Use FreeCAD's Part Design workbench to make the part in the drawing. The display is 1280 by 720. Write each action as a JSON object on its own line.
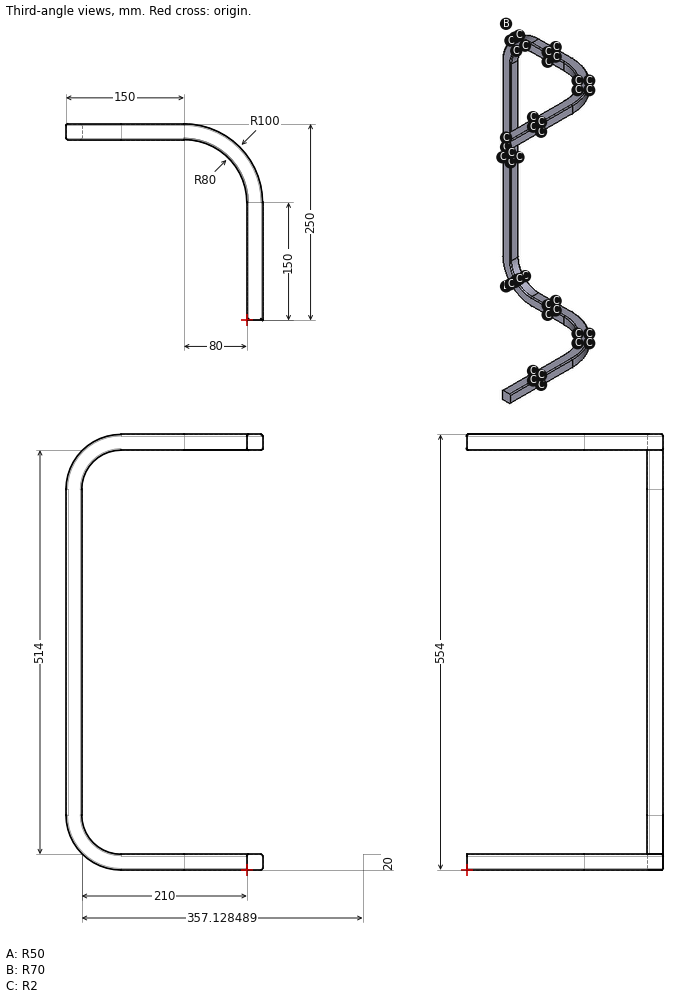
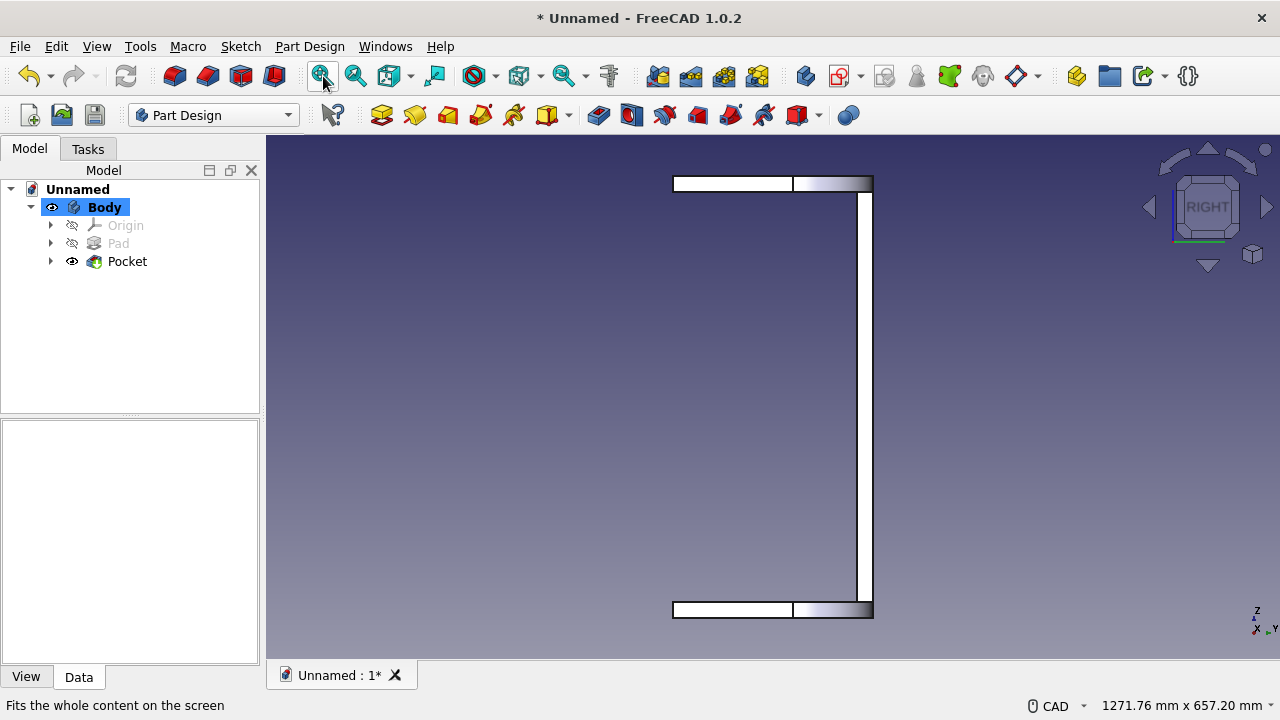
{"action": "key", "text": "5"}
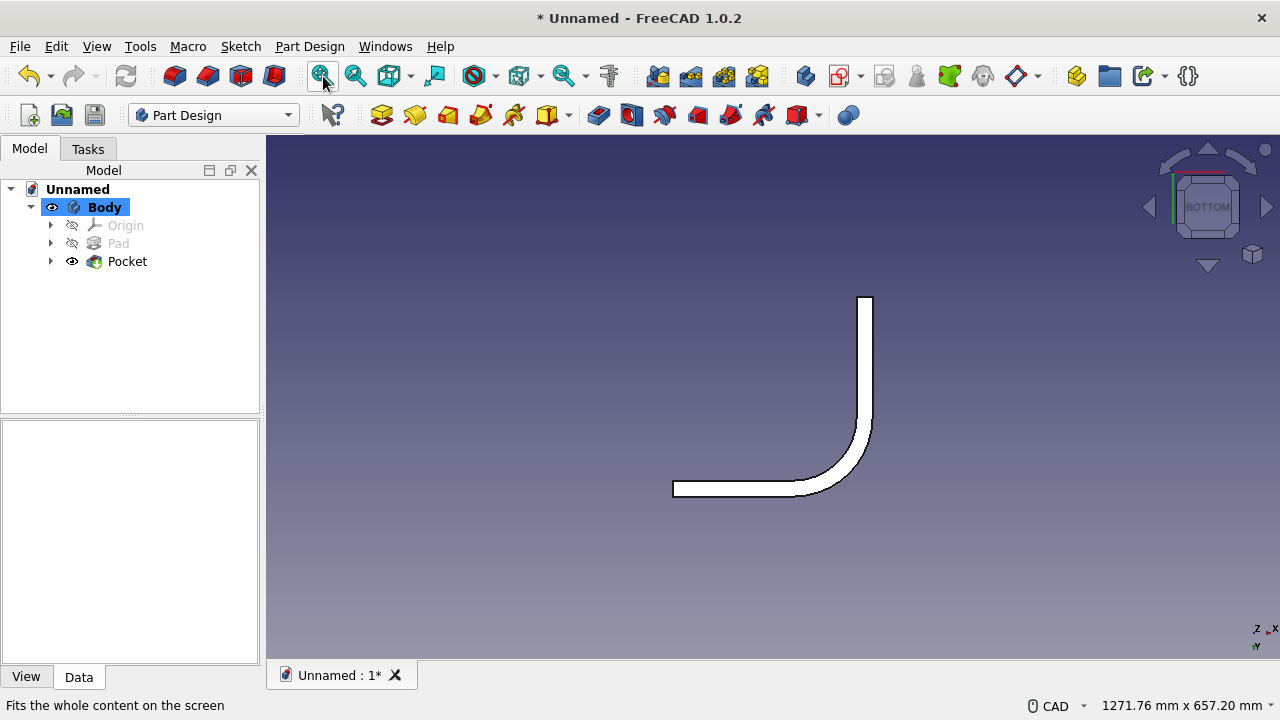
{"action": "left_click", "coordinate": [323, 76]}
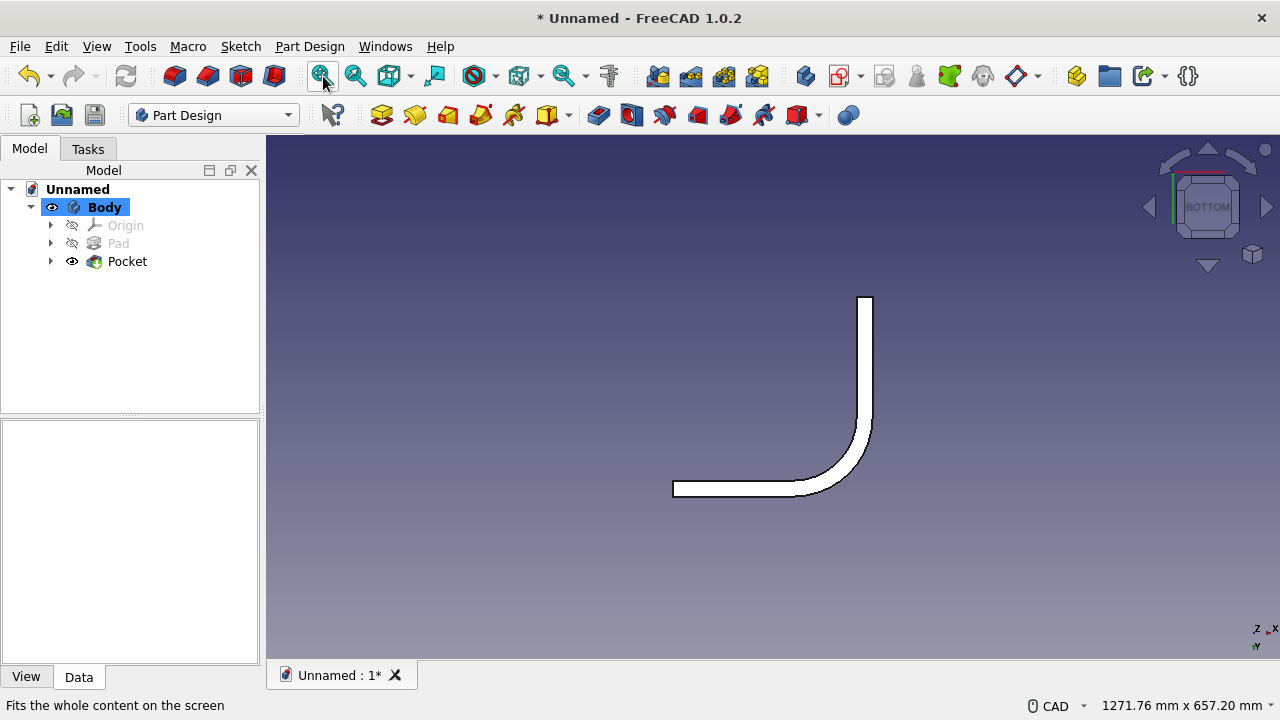
{"action": "scroll", "coordinate": [689, 488], "scroll_direction": "up", "scroll_amount": 5}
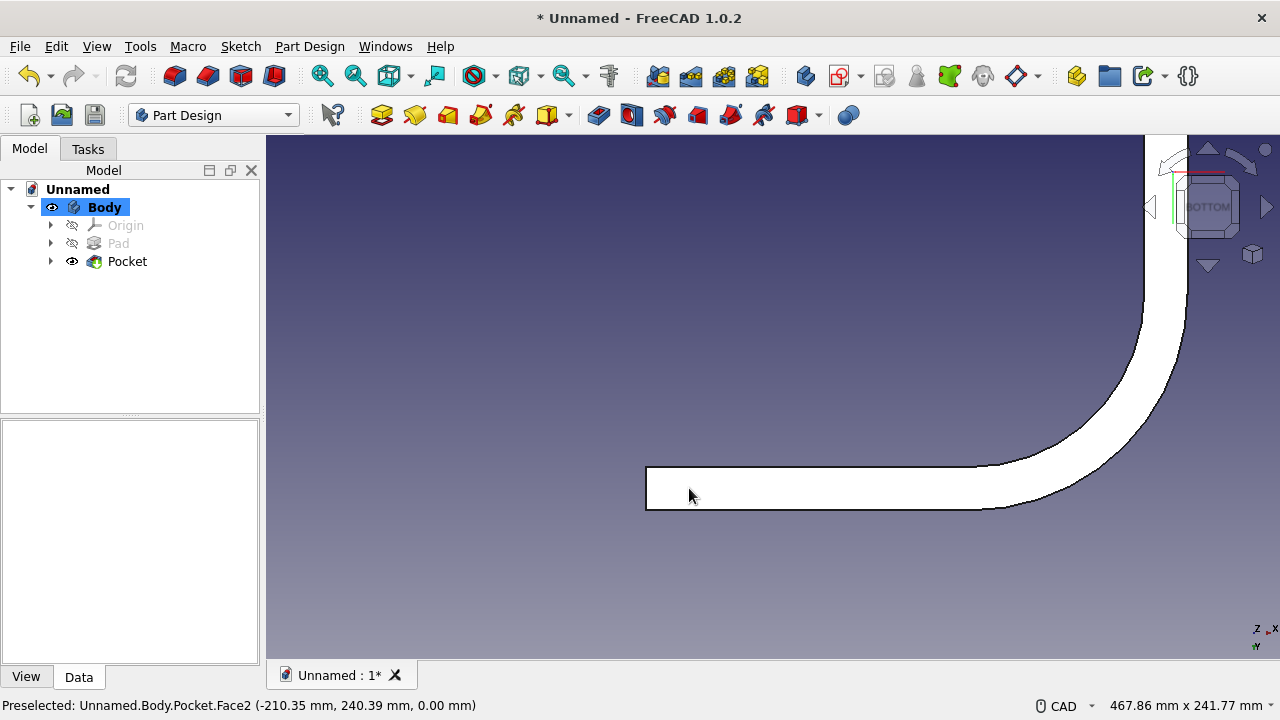
{"action": "left_click", "coordinate": [323, 76]}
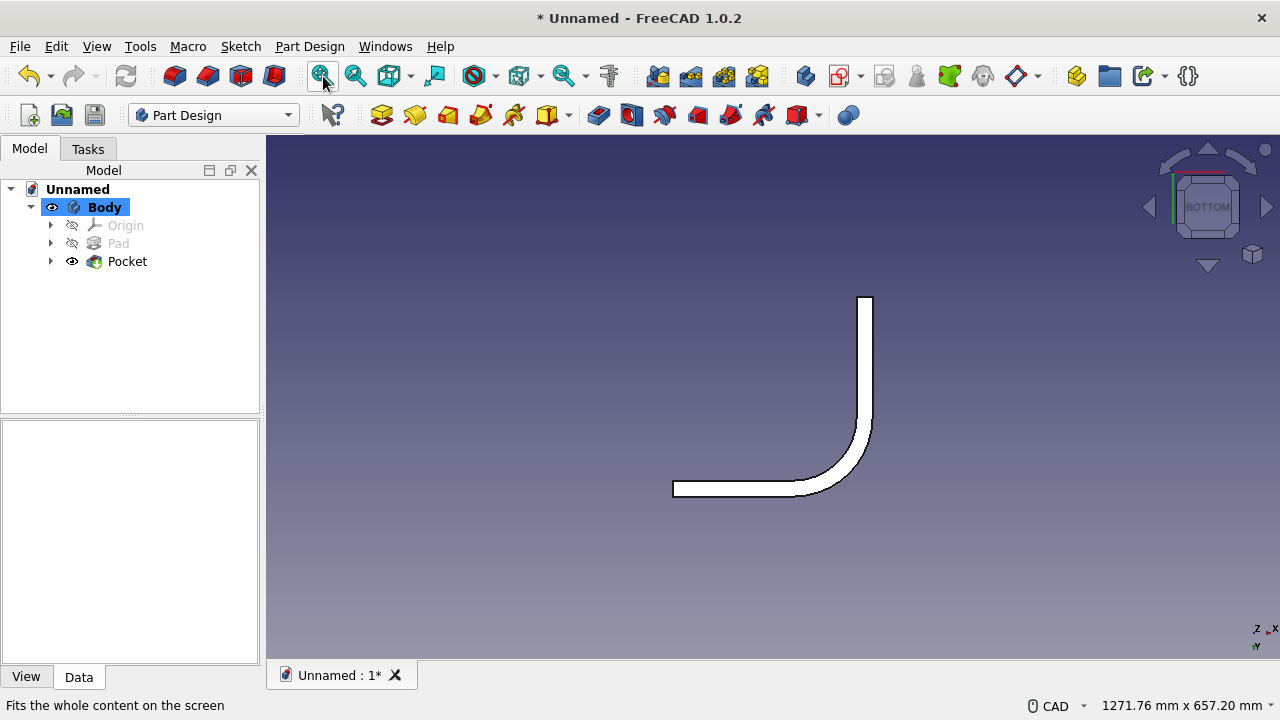
{"action": "key", "text": "4"}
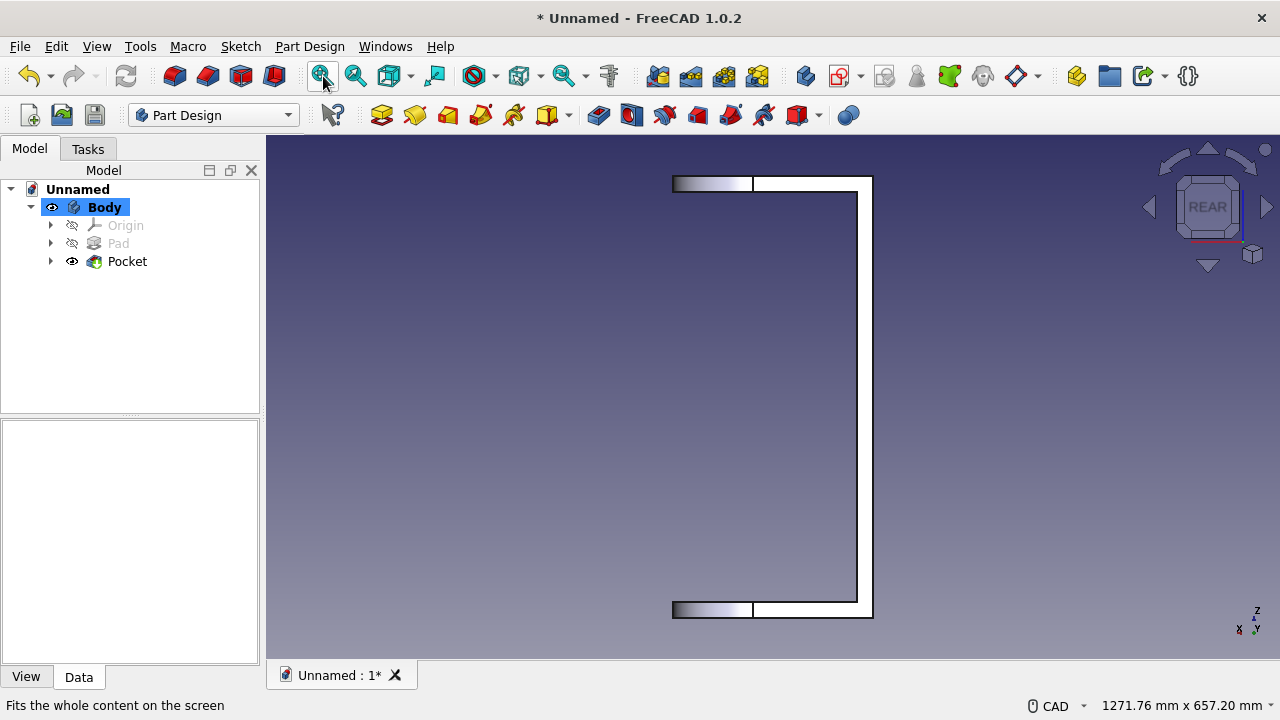
{"action": "scroll", "coordinate": [857, 191], "scroll_direction": "up", "scroll_amount": 5}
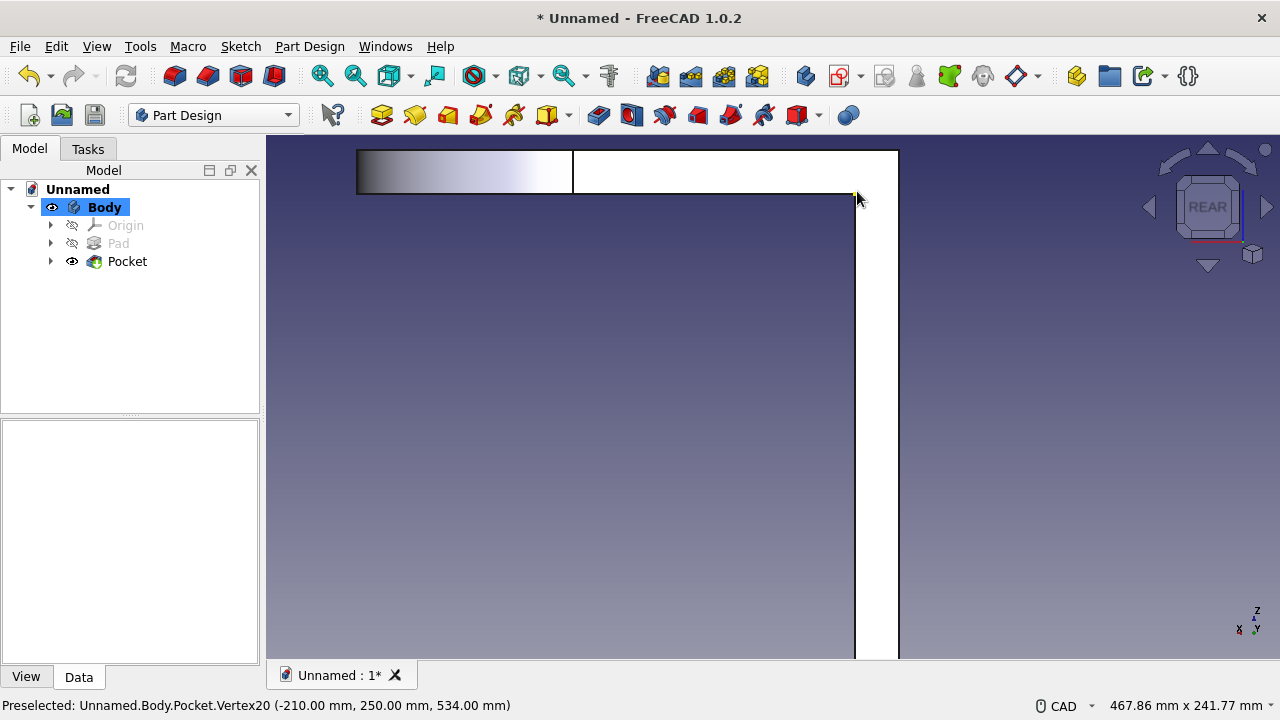
{"action": "left_click", "coordinate": [323, 76]}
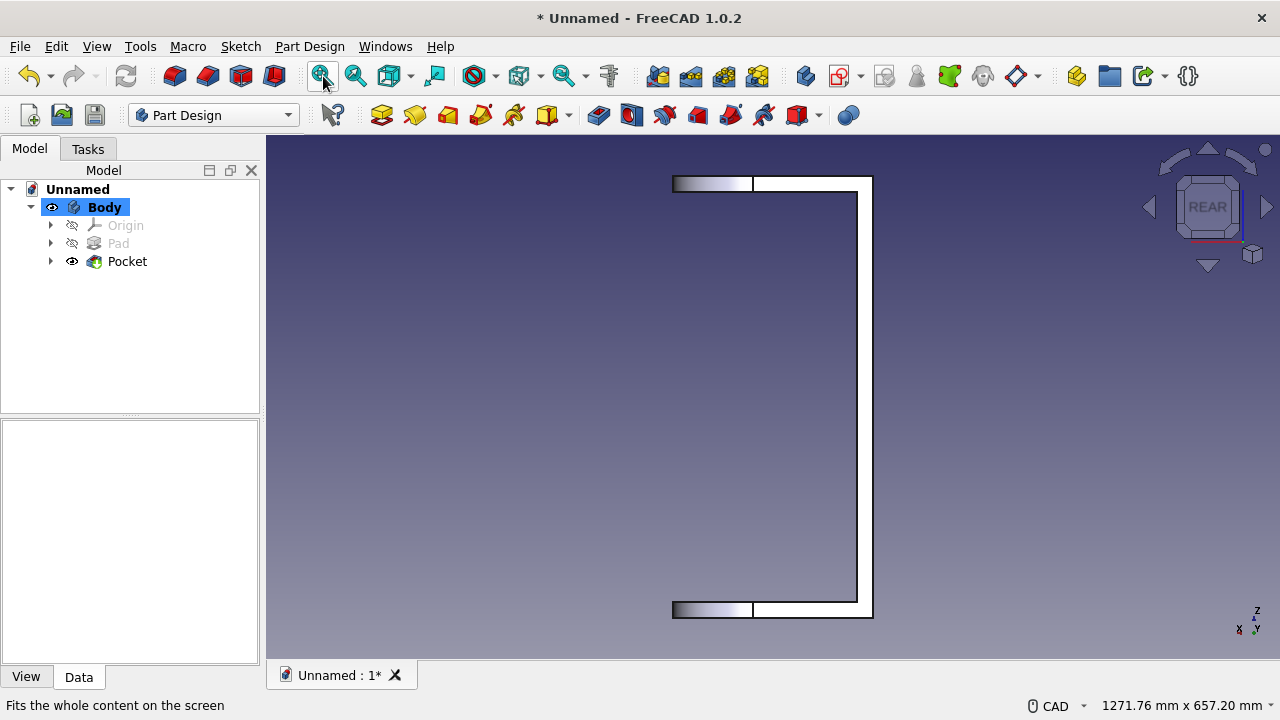
{"action": "key", "text": "6"}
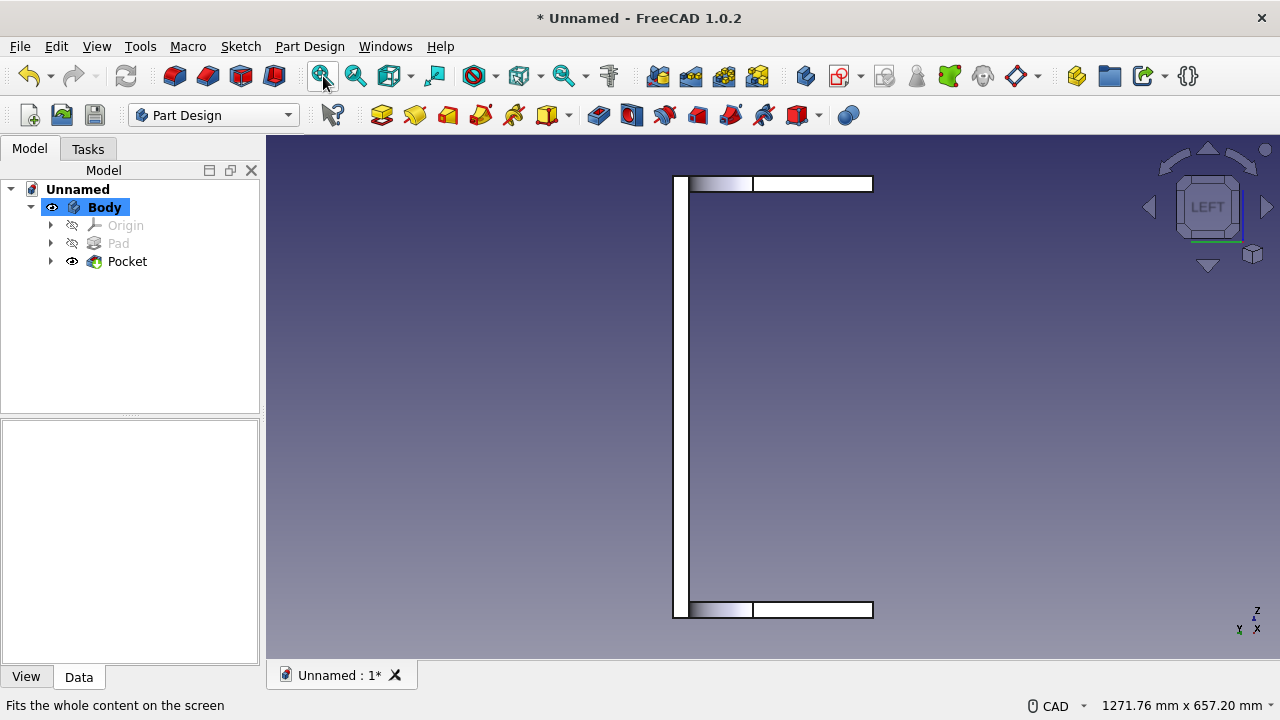
{"action": "scroll", "coordinate": [681, 191], "scroll_direction": "up", "scroll_amount": 5}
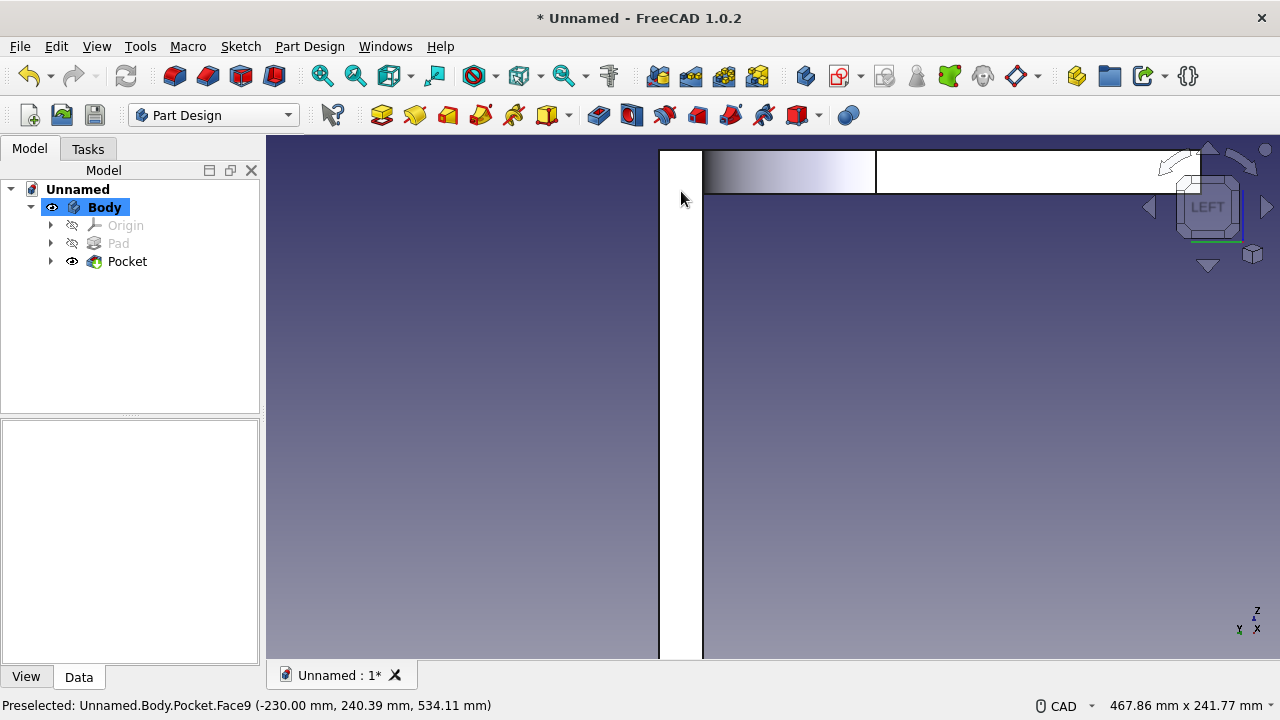
{"action": "left_click", "coordinate": [323, 76]}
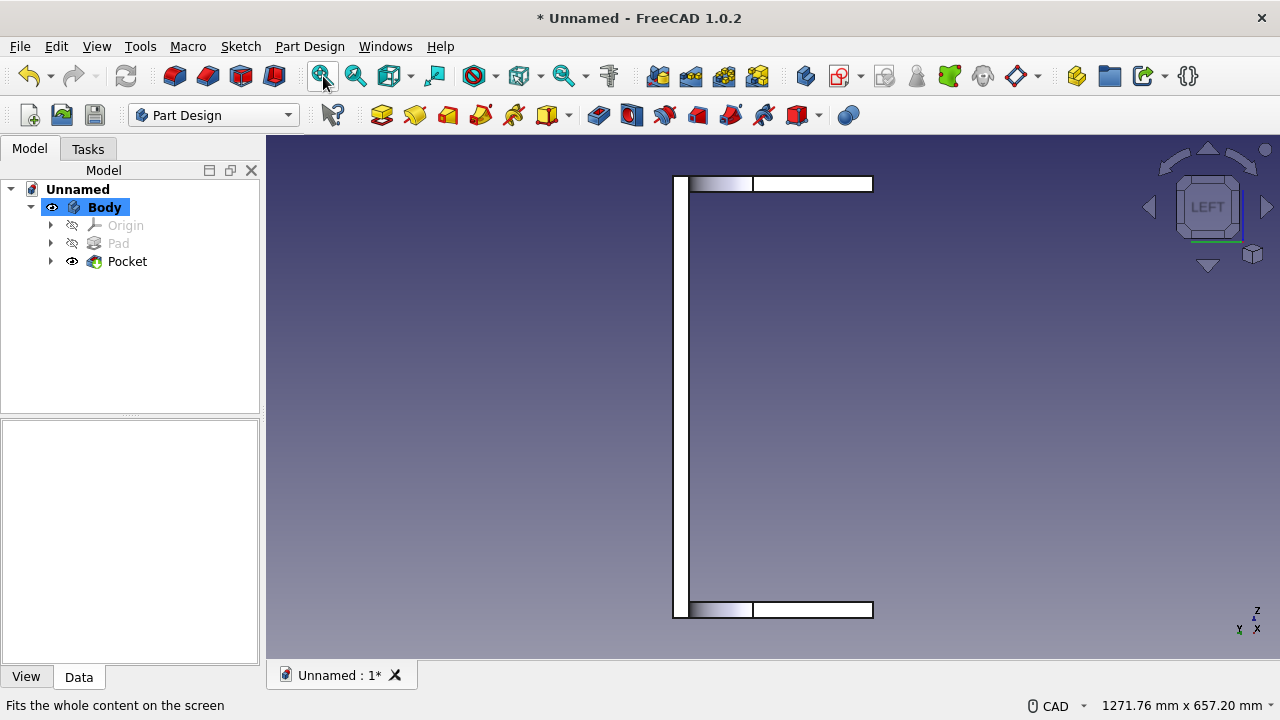
{"action": "key", "text": "v 3"}